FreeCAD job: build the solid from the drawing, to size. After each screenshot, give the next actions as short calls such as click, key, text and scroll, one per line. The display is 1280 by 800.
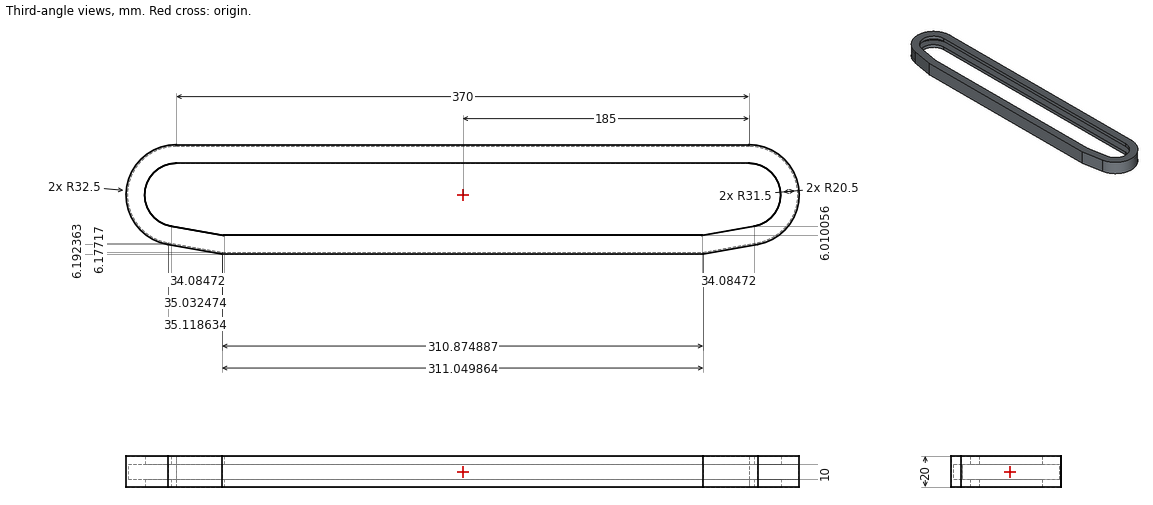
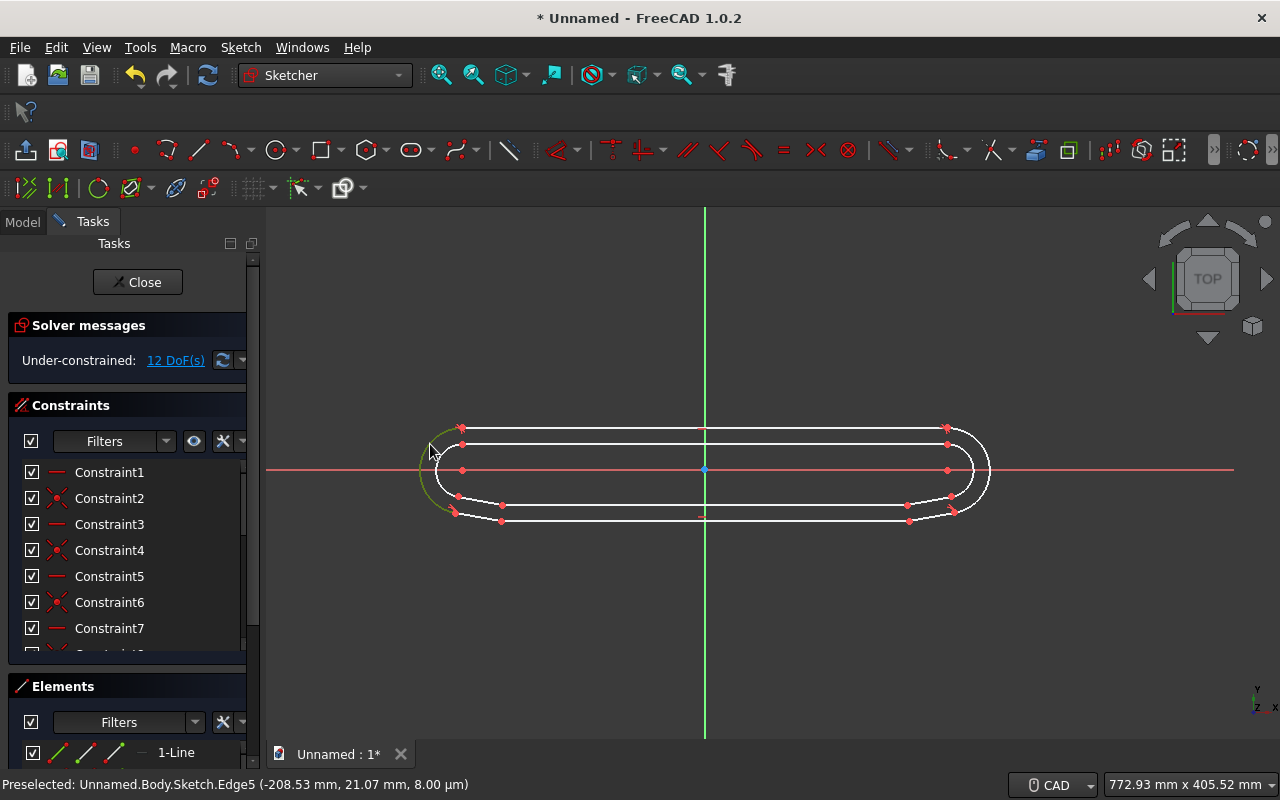
click(984, 492)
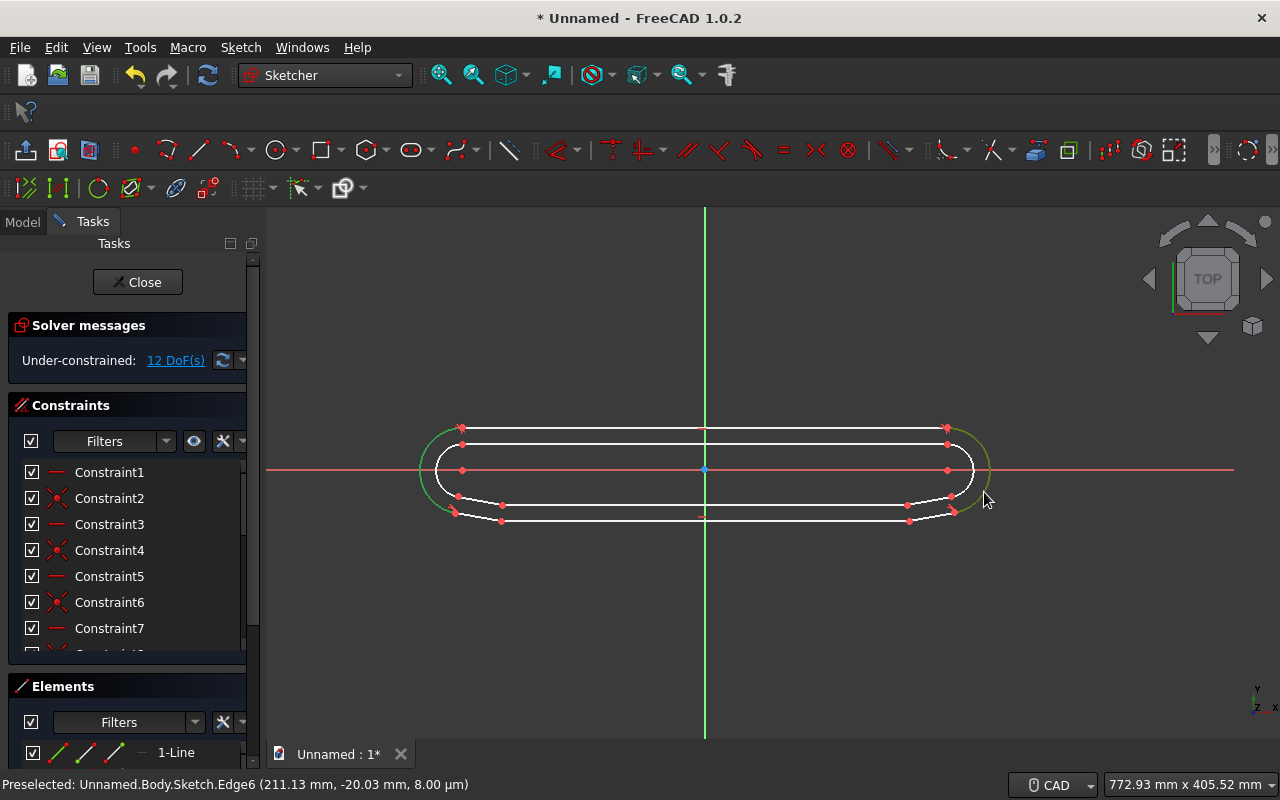
key(e)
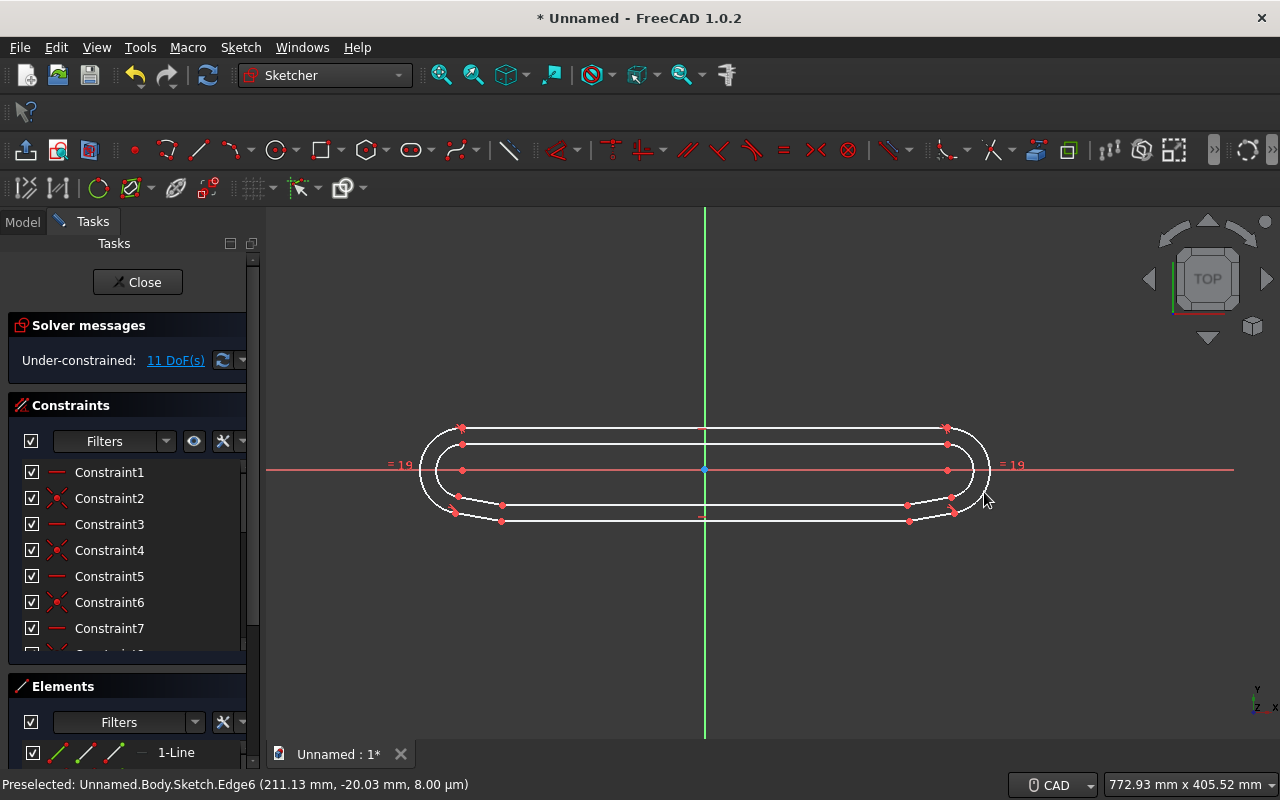
click(463, 471)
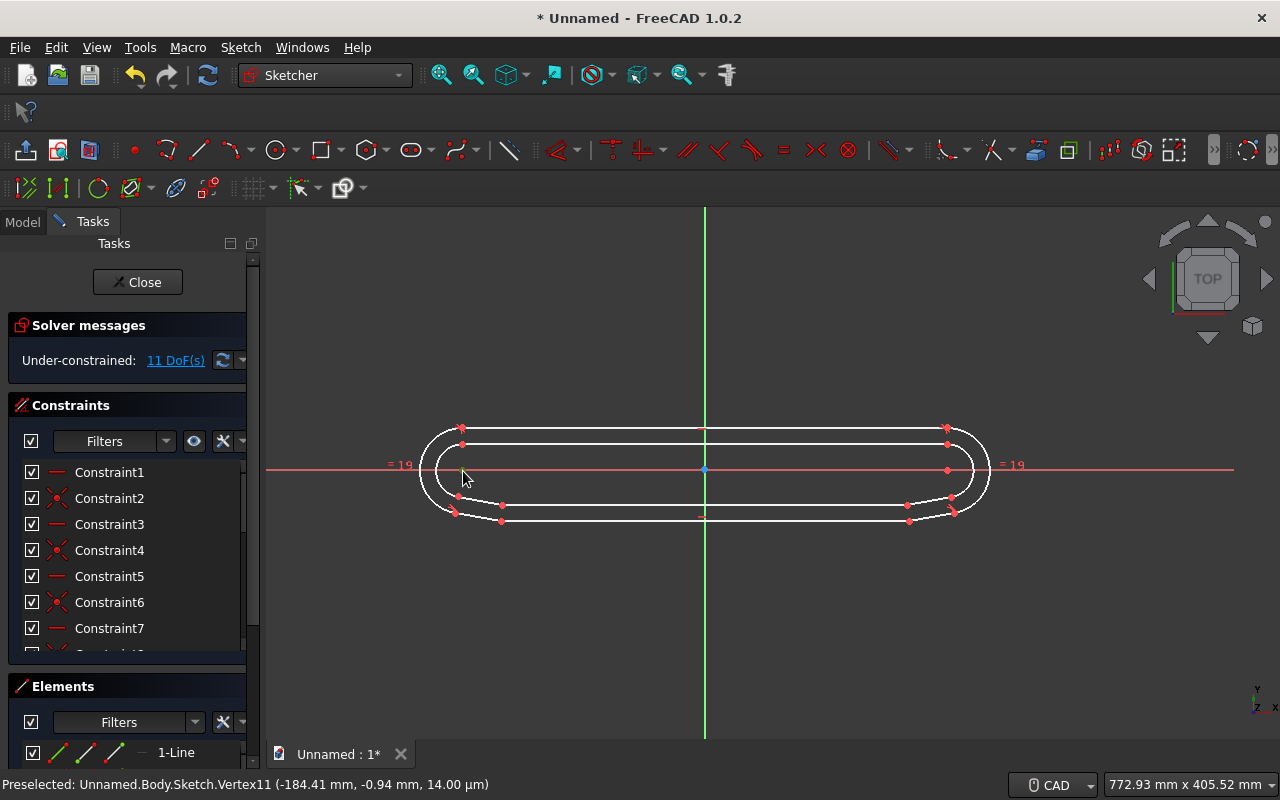
click(353, 470)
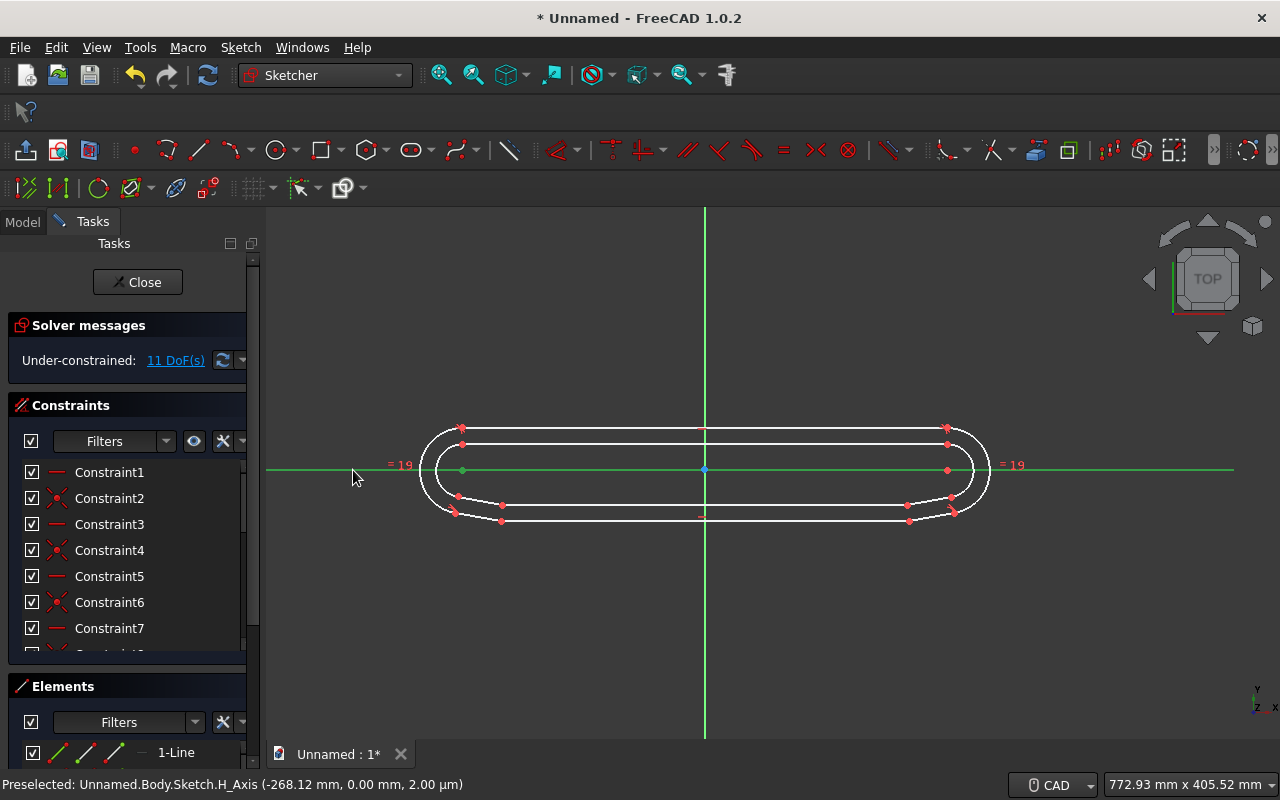
click(612, 150)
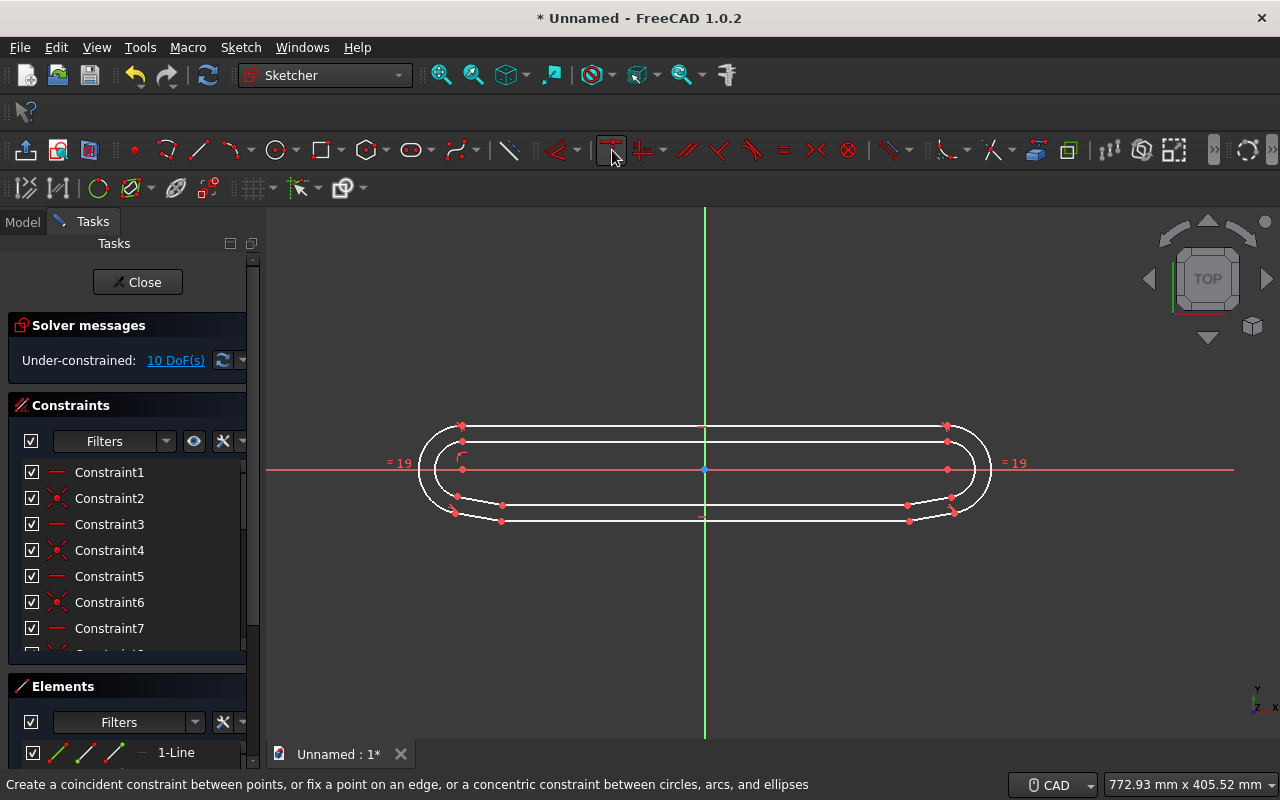
click(429, 442)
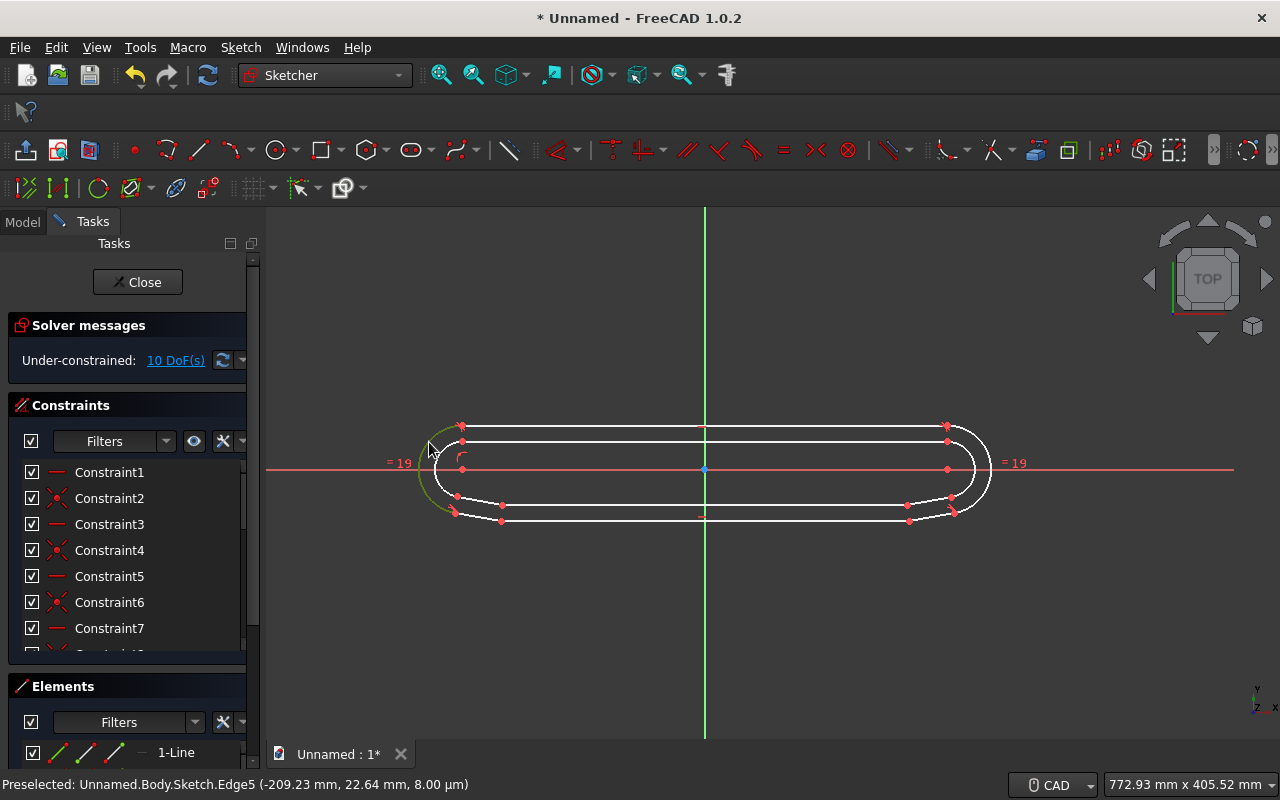
key(k)
key(r)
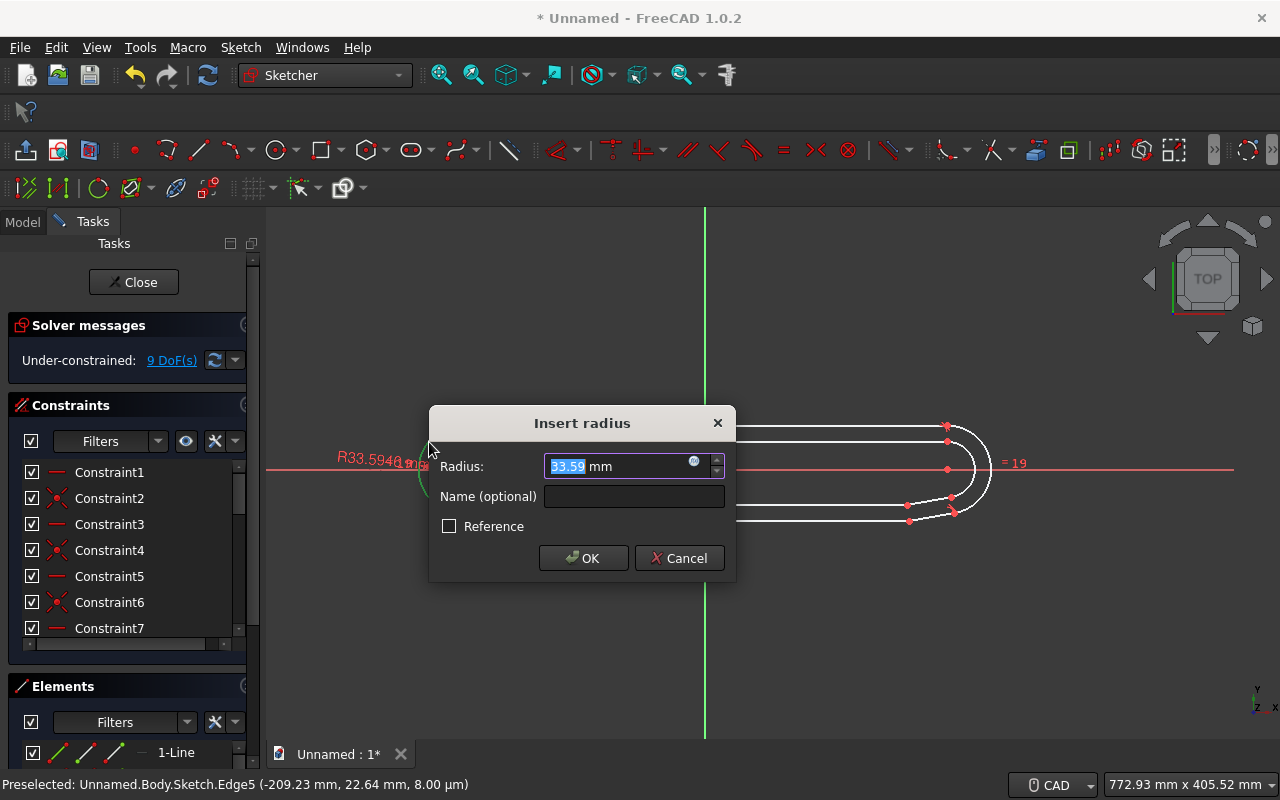
text(32.5)
key(Return)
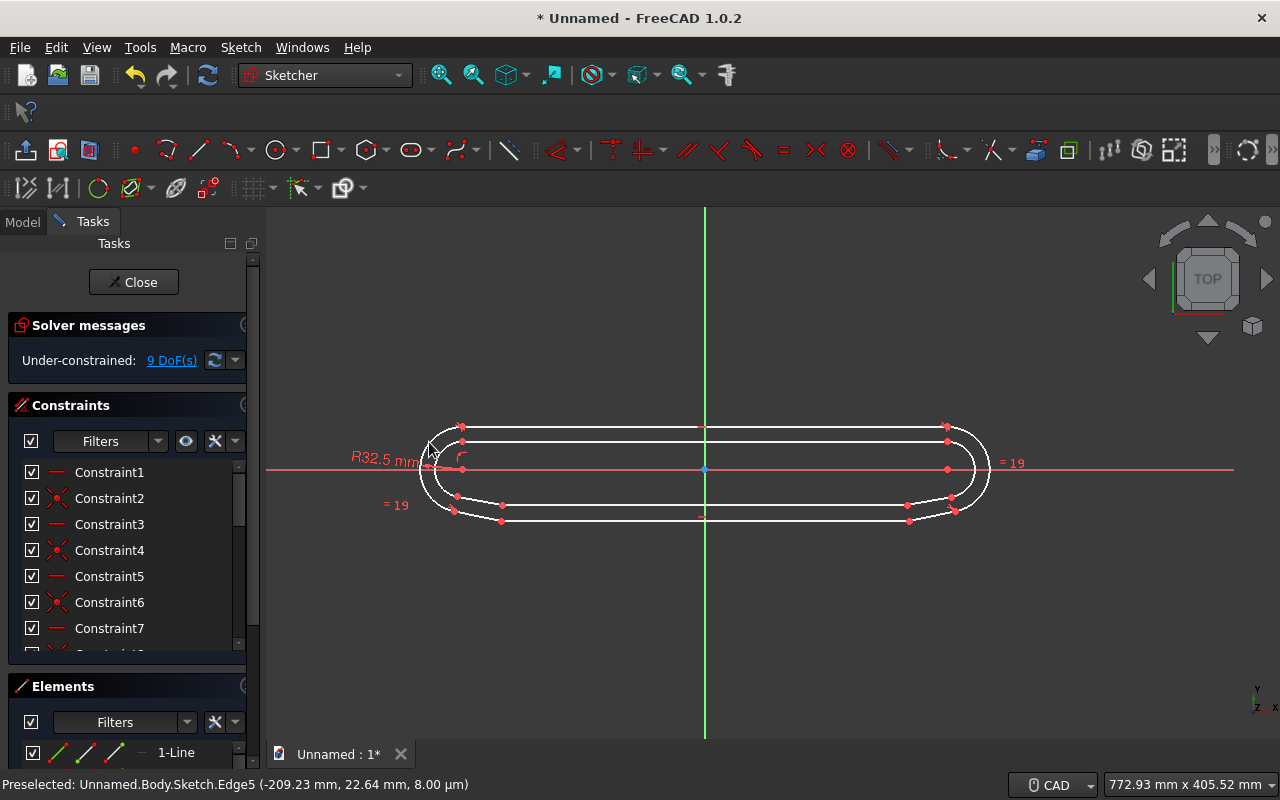
scroll(971, 483, up, 2)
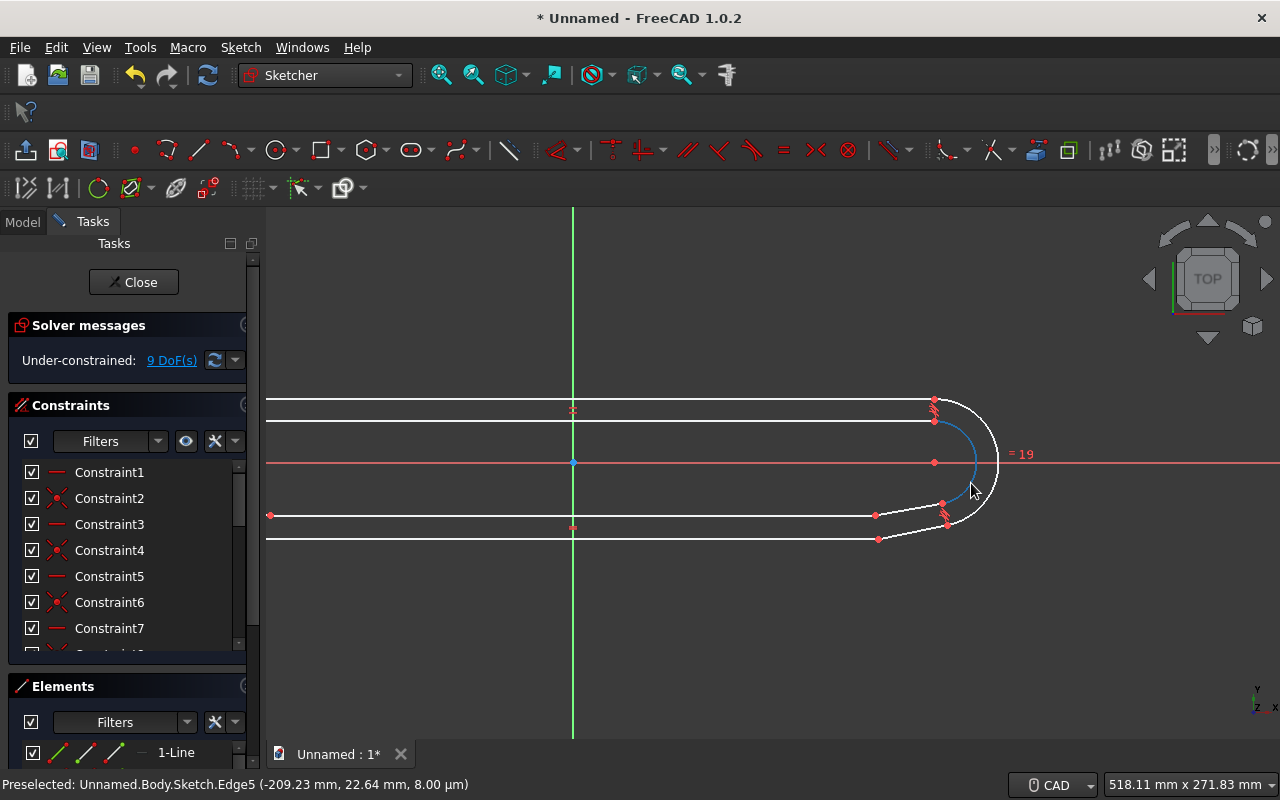
click(971, 483)